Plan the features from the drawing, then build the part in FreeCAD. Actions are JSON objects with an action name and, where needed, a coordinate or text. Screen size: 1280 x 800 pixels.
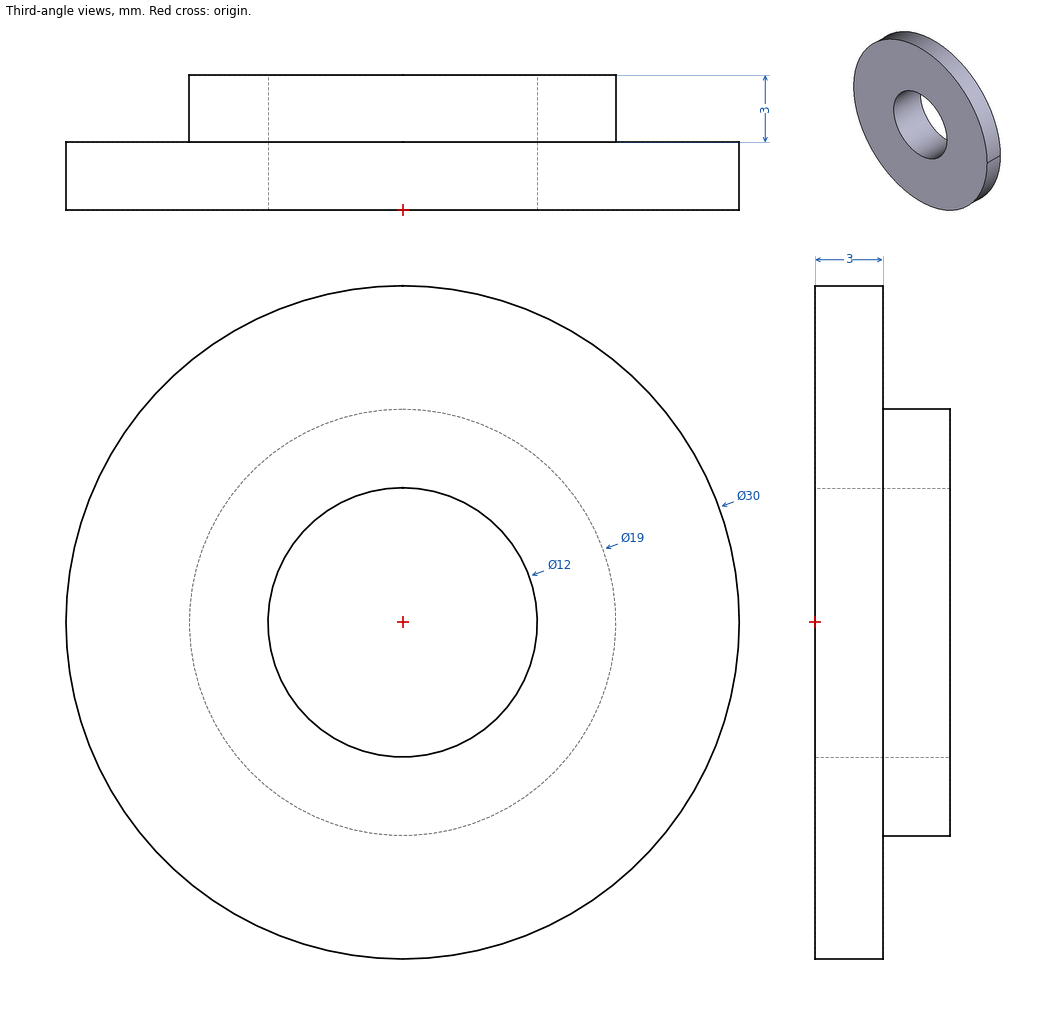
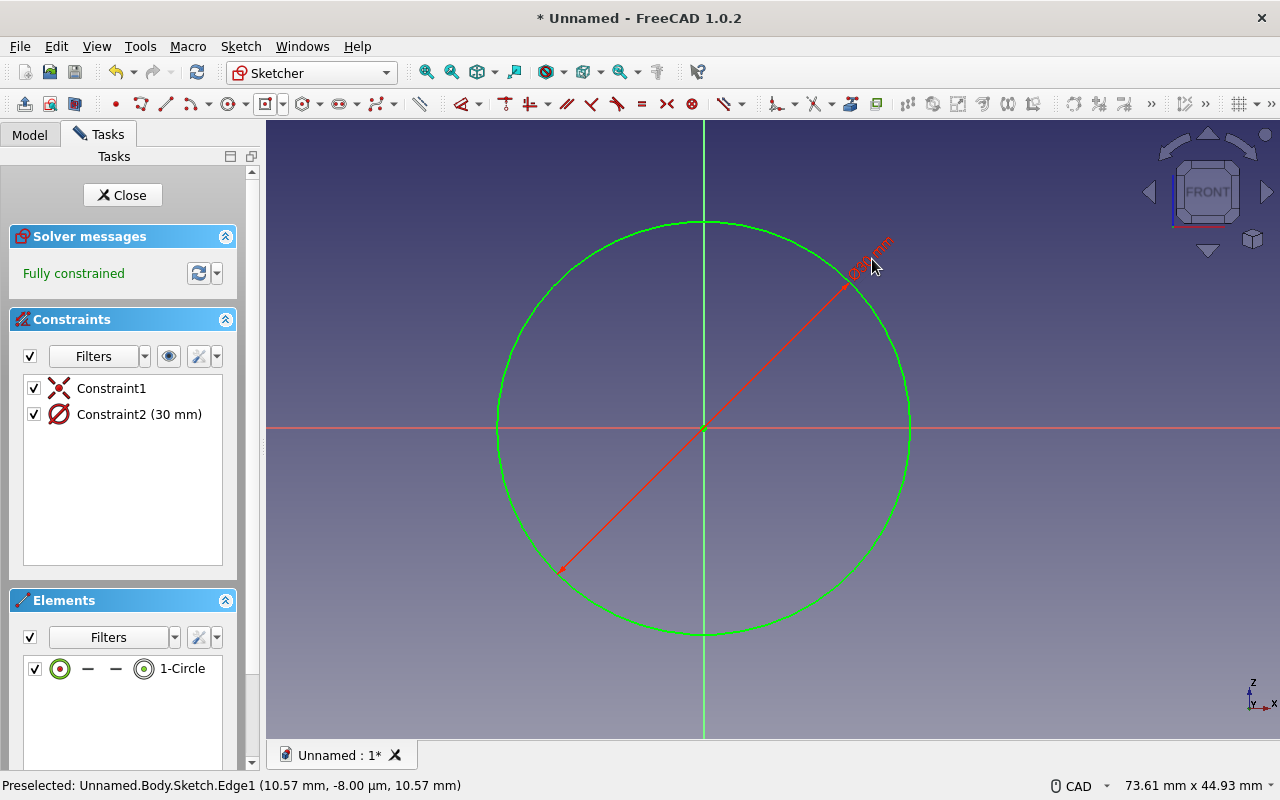
{"action": "left_click", "coordinate": [123, 195]}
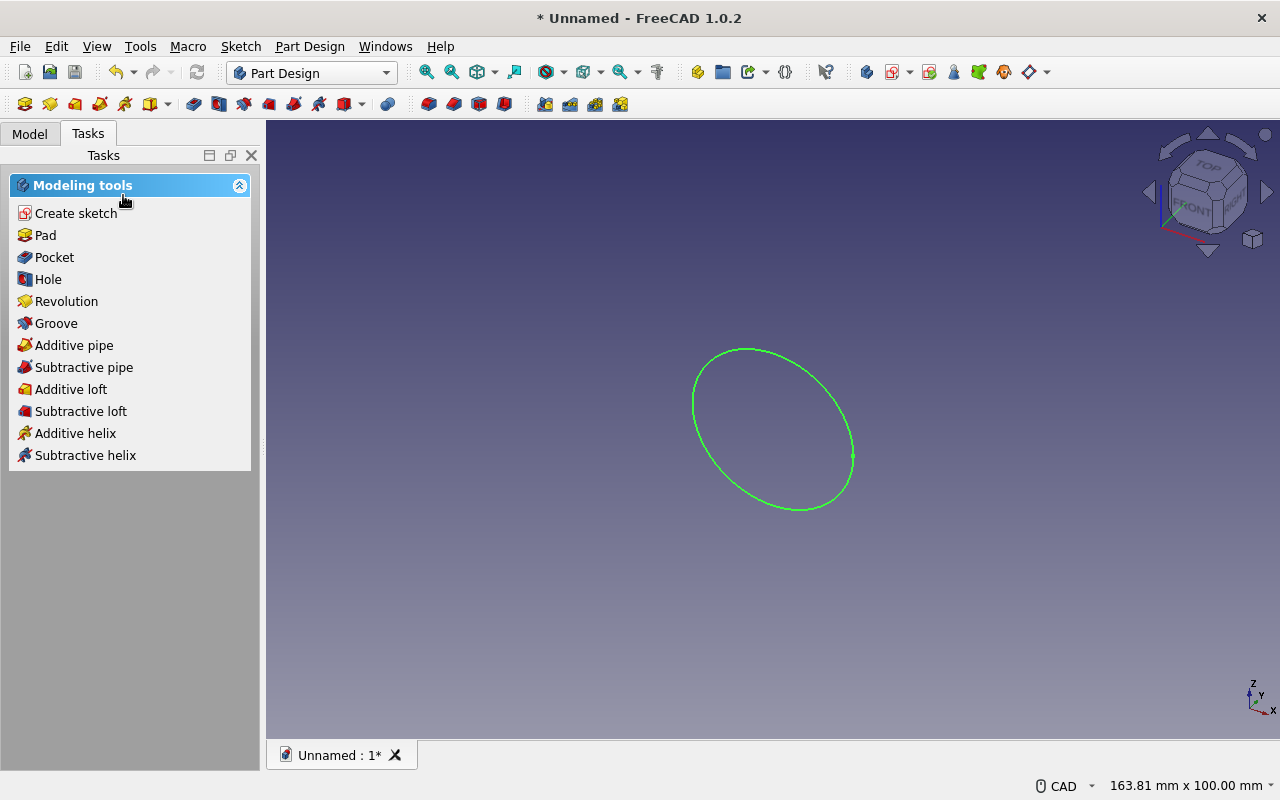
{"action": "left_click", "coordinate": [25, 104]}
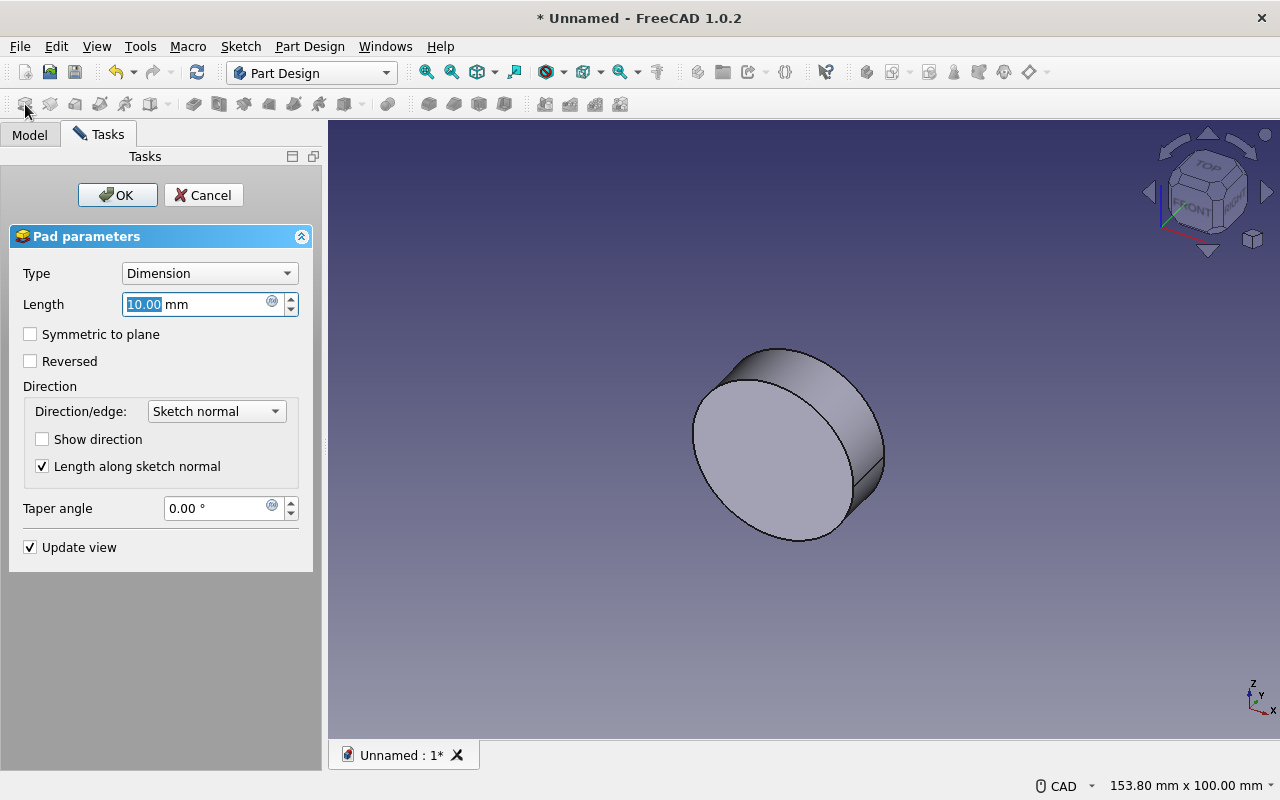
{"action": "type", "text": "3"}
{"action": "key", "text": "Tab"}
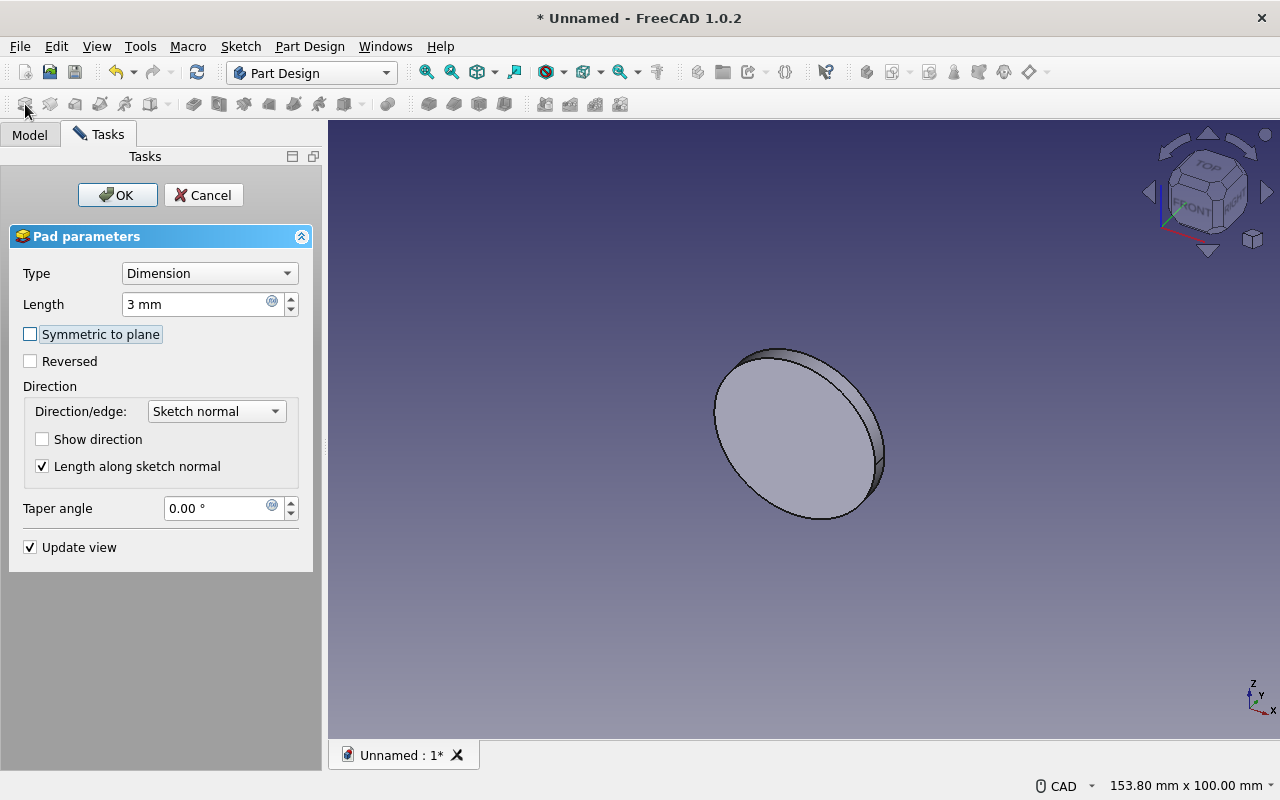
{"action": "left_click", "coordinate": [31, 361]}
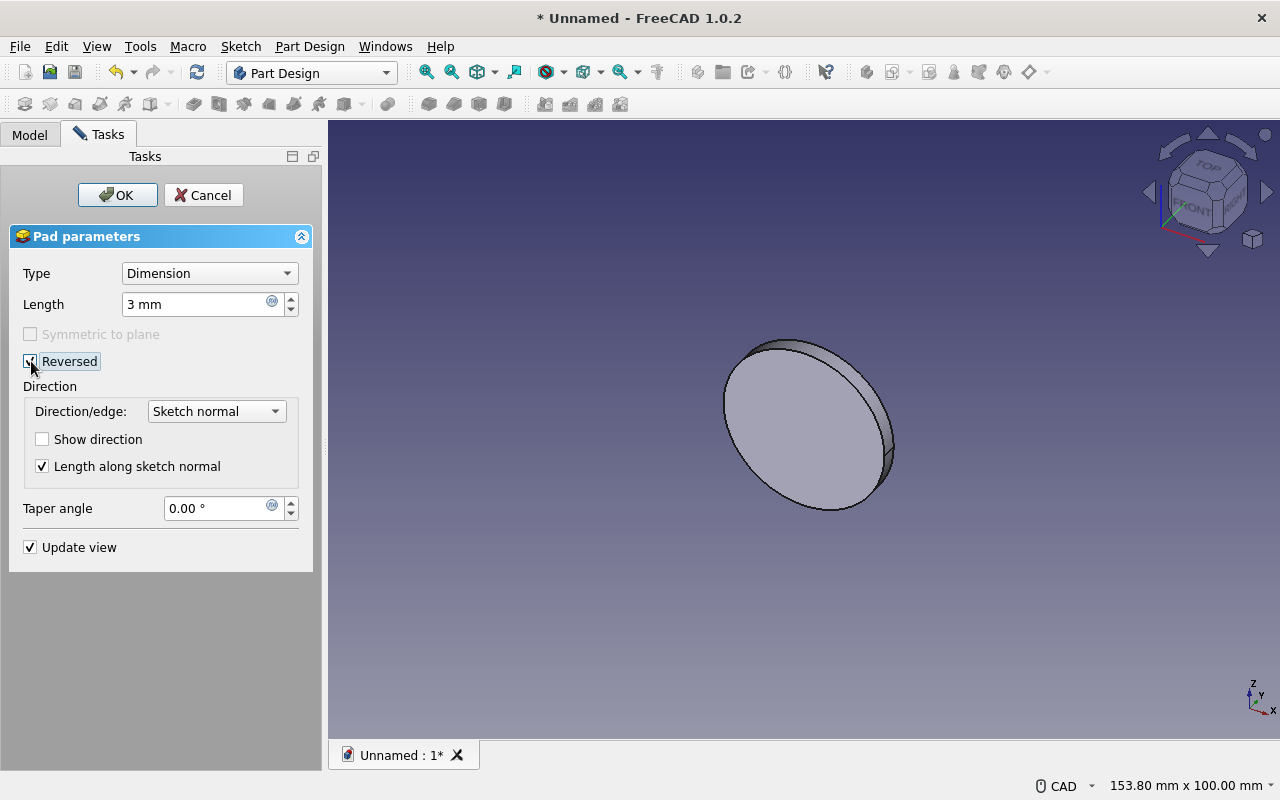
{"action": "left_click", "coordinate": [118, 195]}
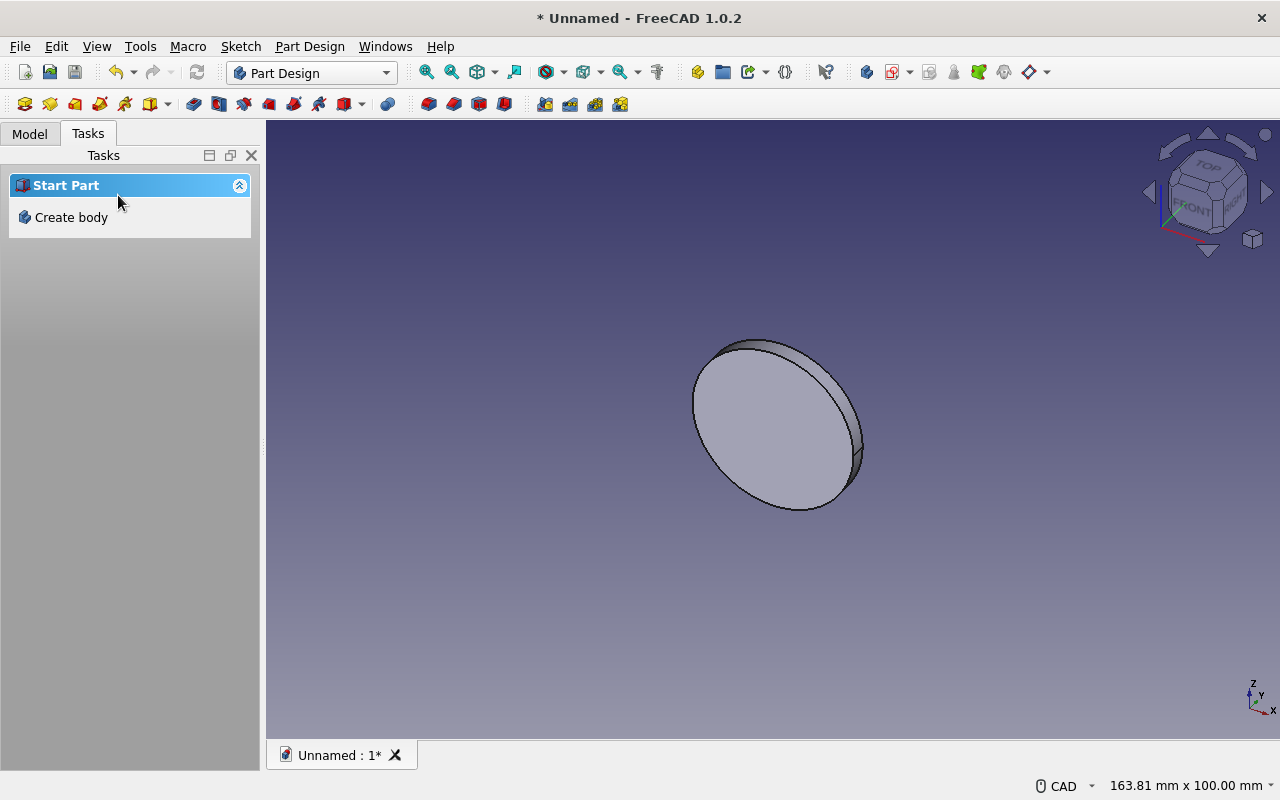
{"action": "left_click", "coordinate": [427, 72]}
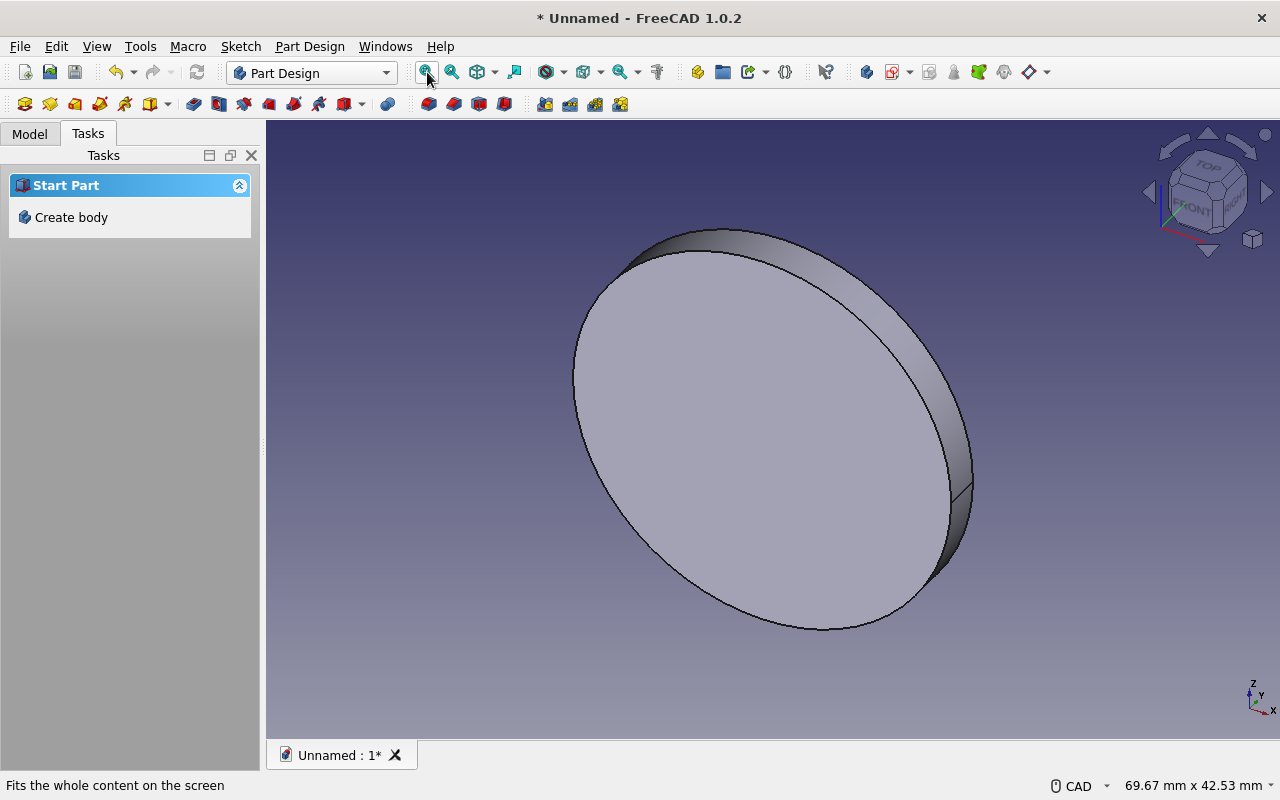
{"action": "key", "text": "4"}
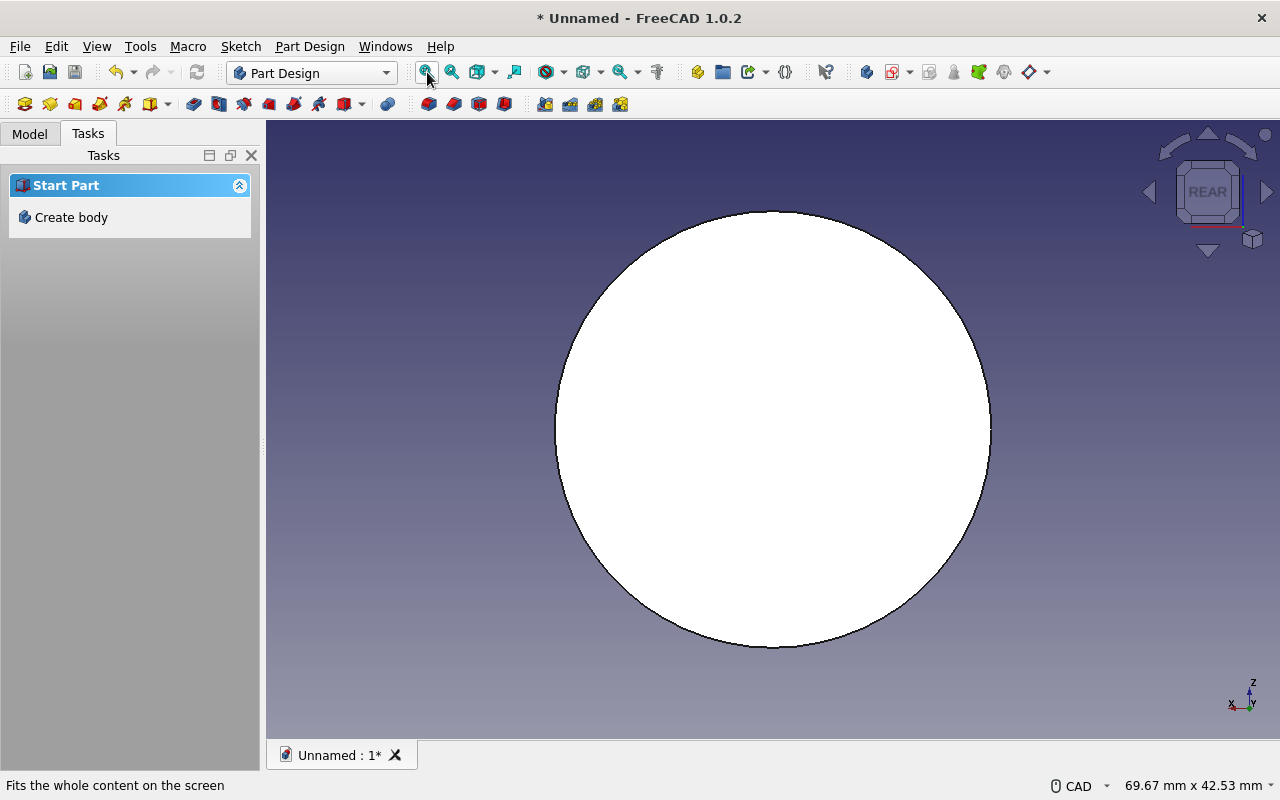
{"action": "left_click", "coordinate": [773, 428]}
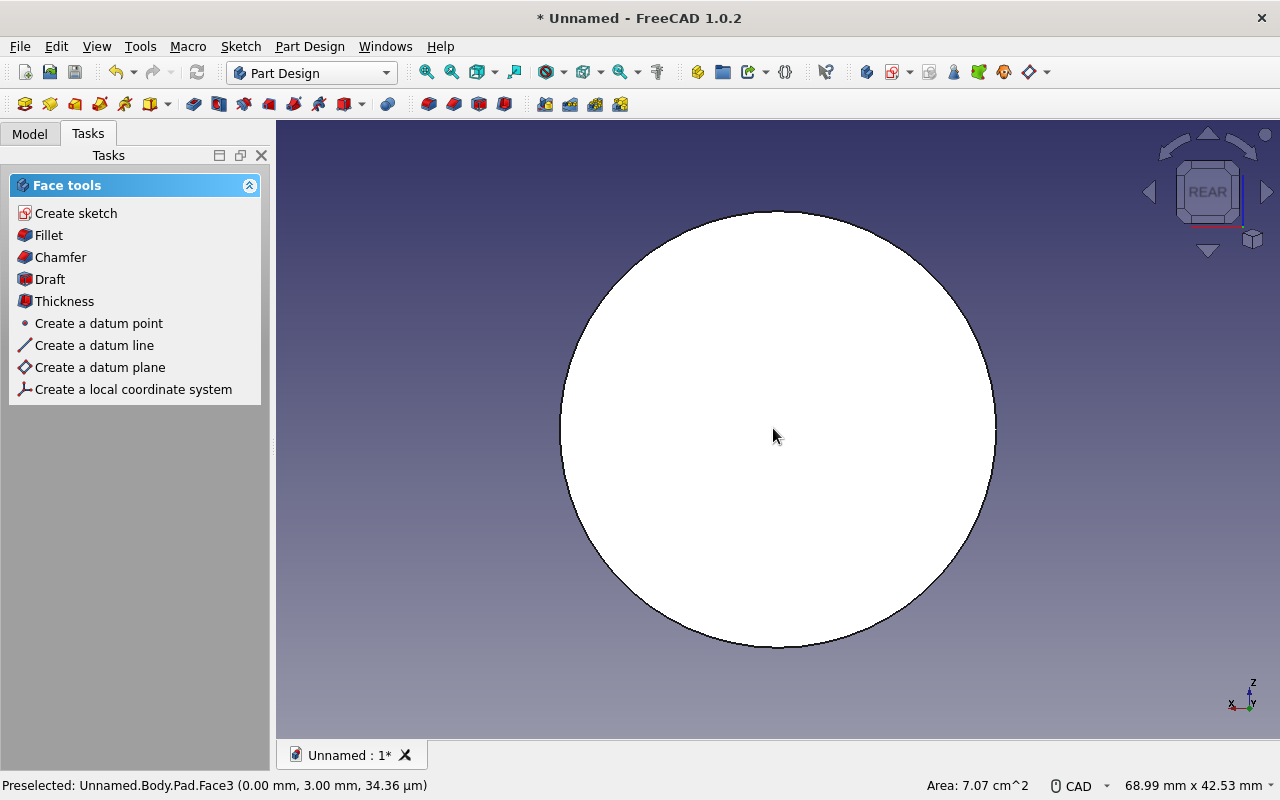
{"action": "left_click", "coordinate": [892, 72]}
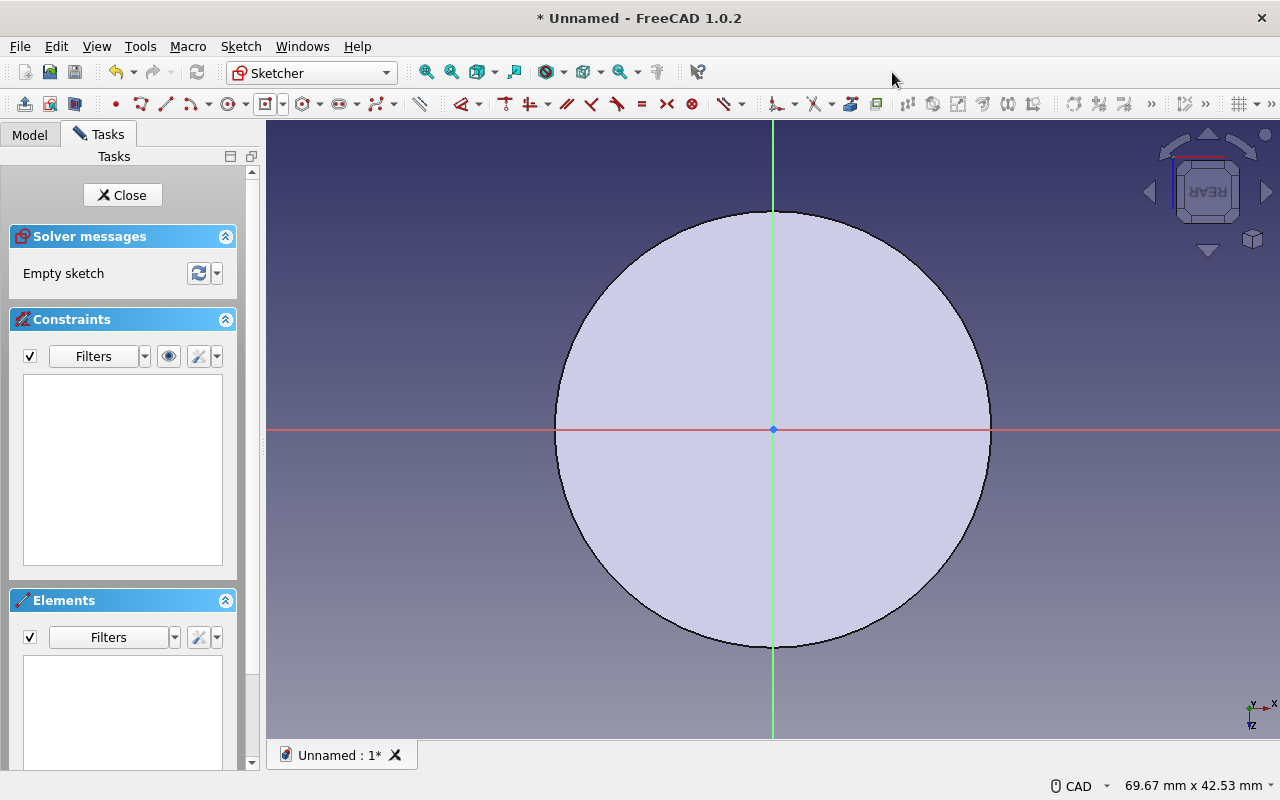
{"action": "scroll", "coordinate": [912, 430], "scroll_direction": "up", "scroll_amount": 2}